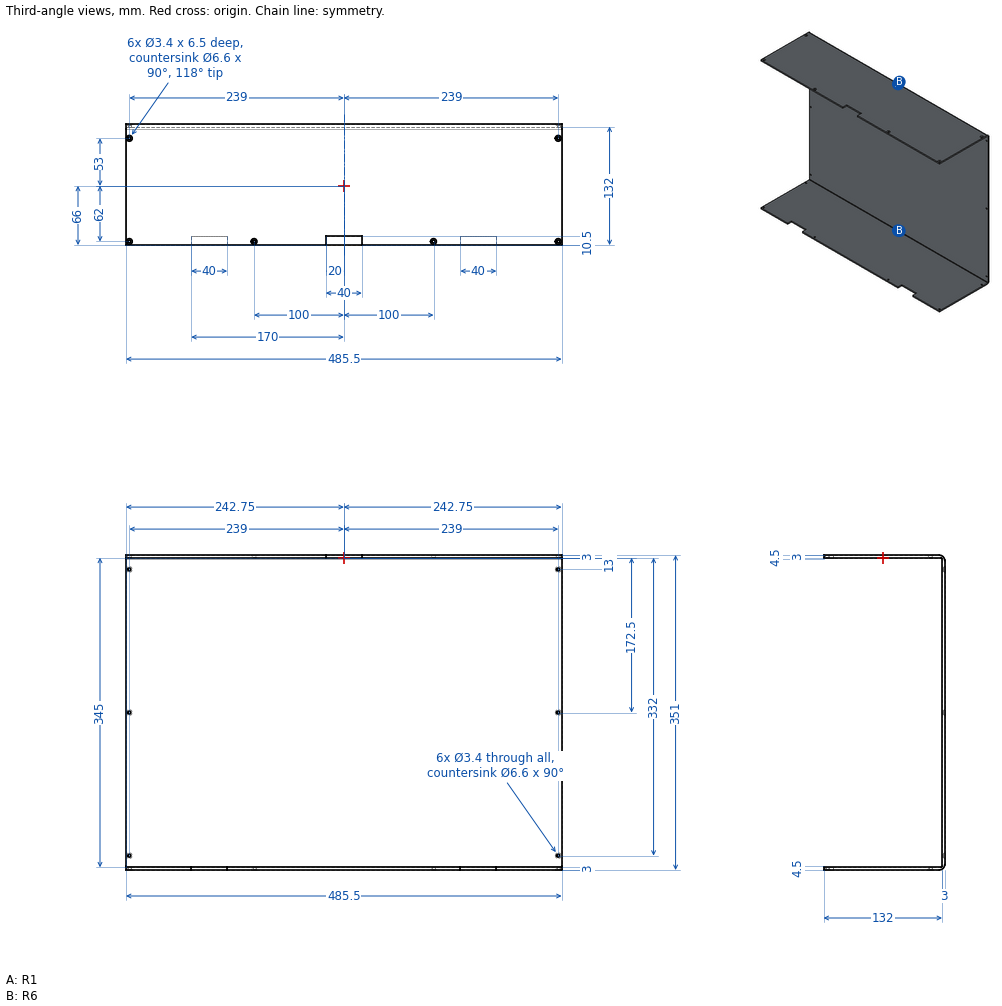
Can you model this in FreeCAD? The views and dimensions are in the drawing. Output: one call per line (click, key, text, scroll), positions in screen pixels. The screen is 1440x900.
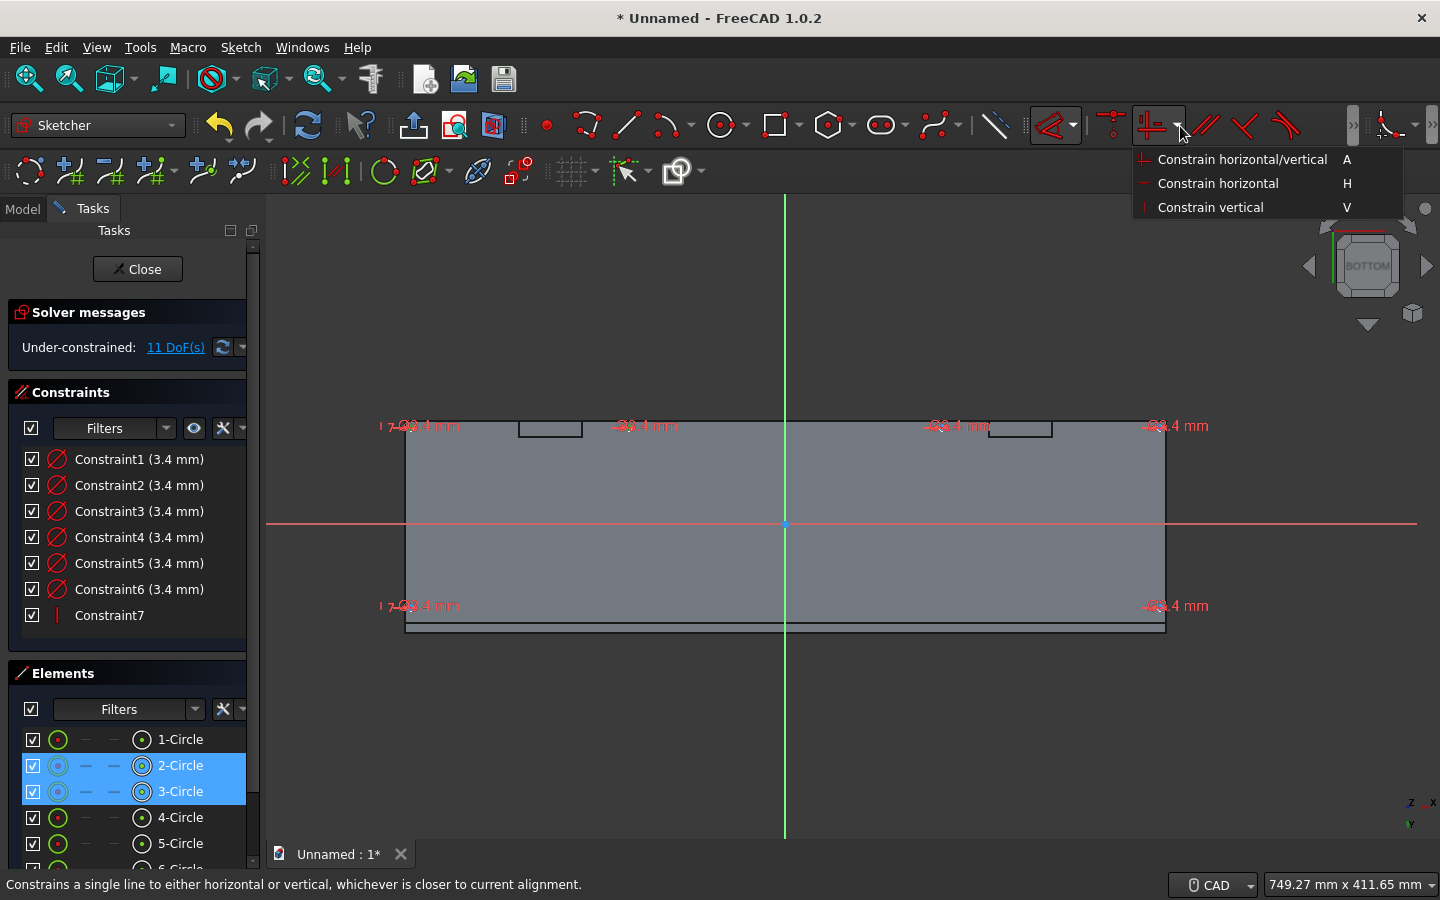
click(1268, 183)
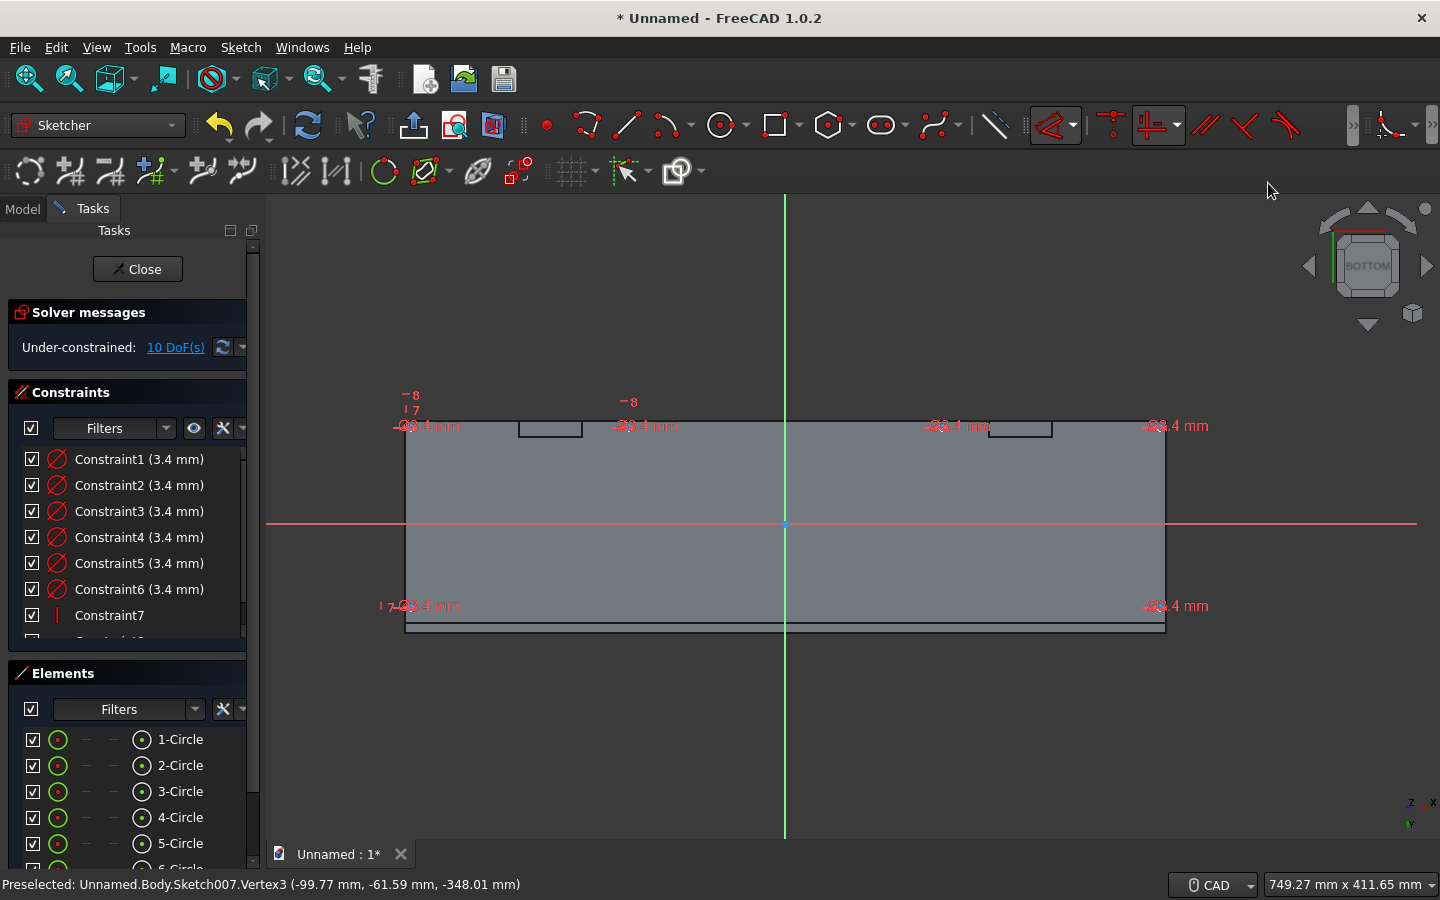
click(629, 428)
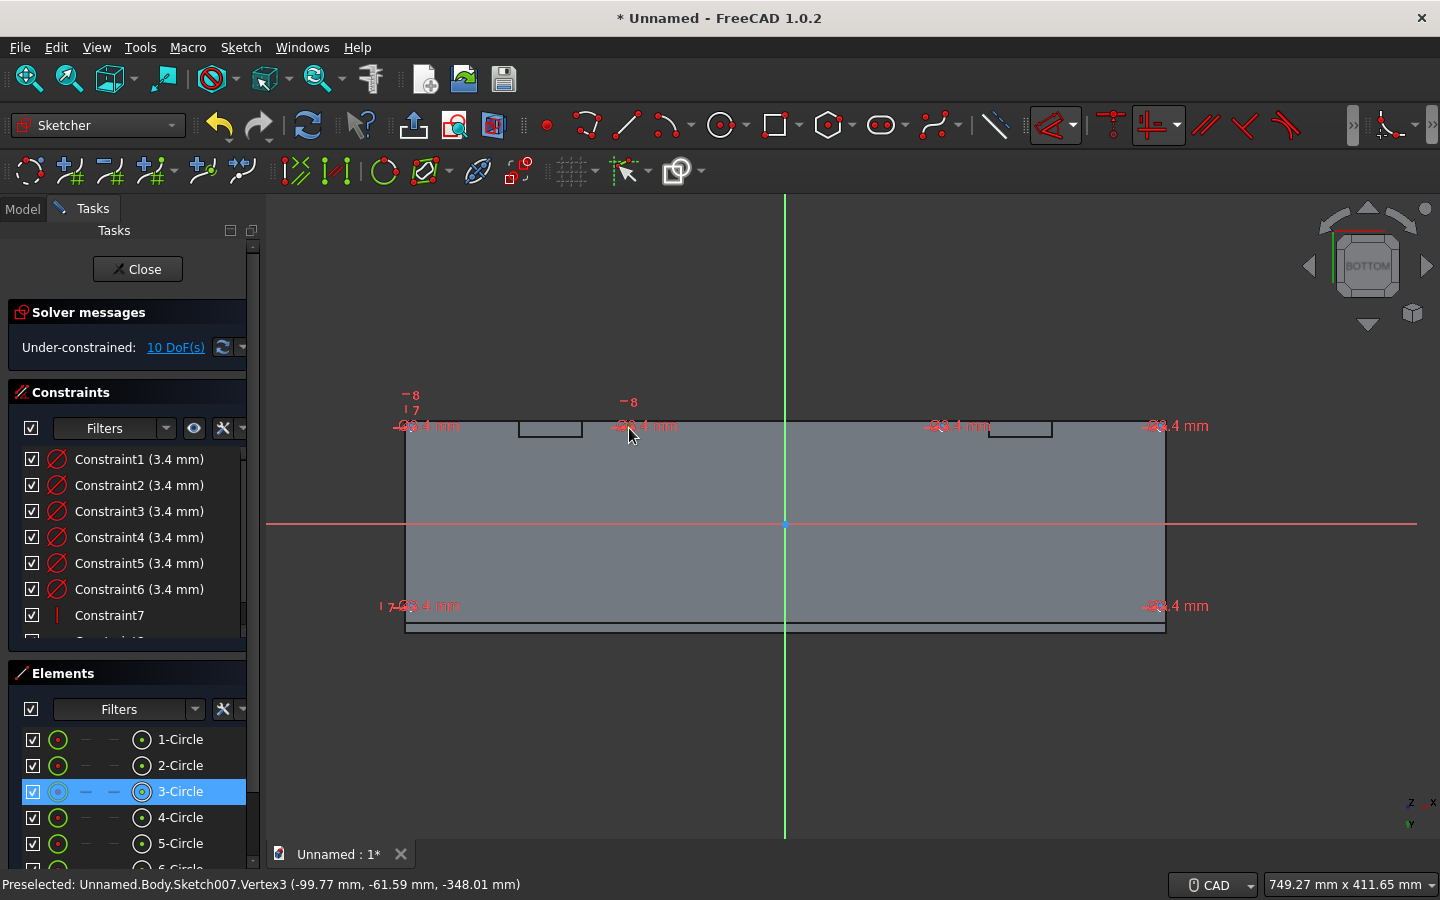
click(942, 428)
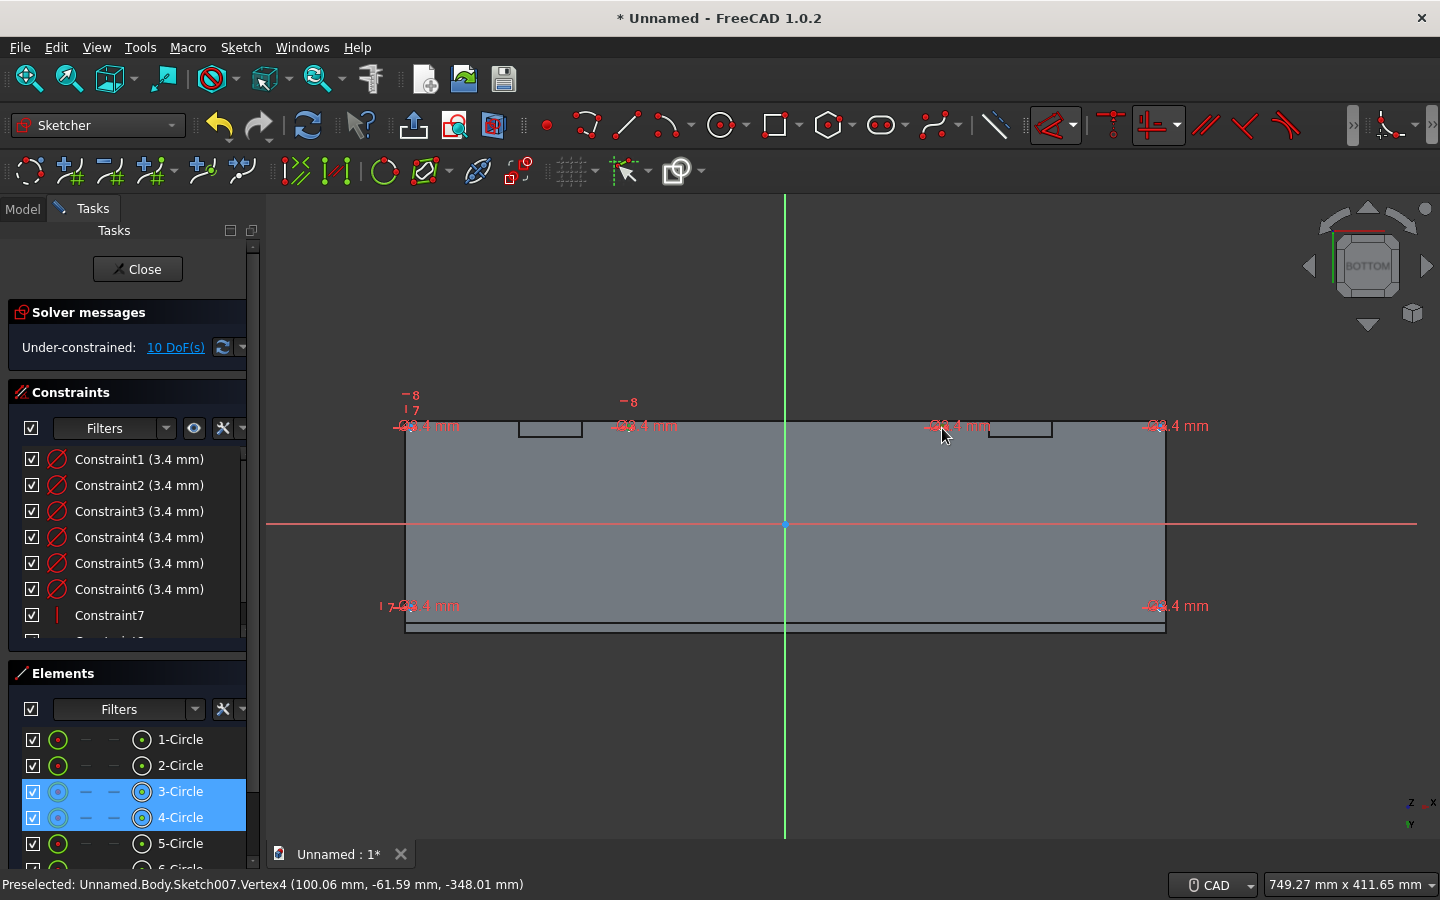
click(1180, 126)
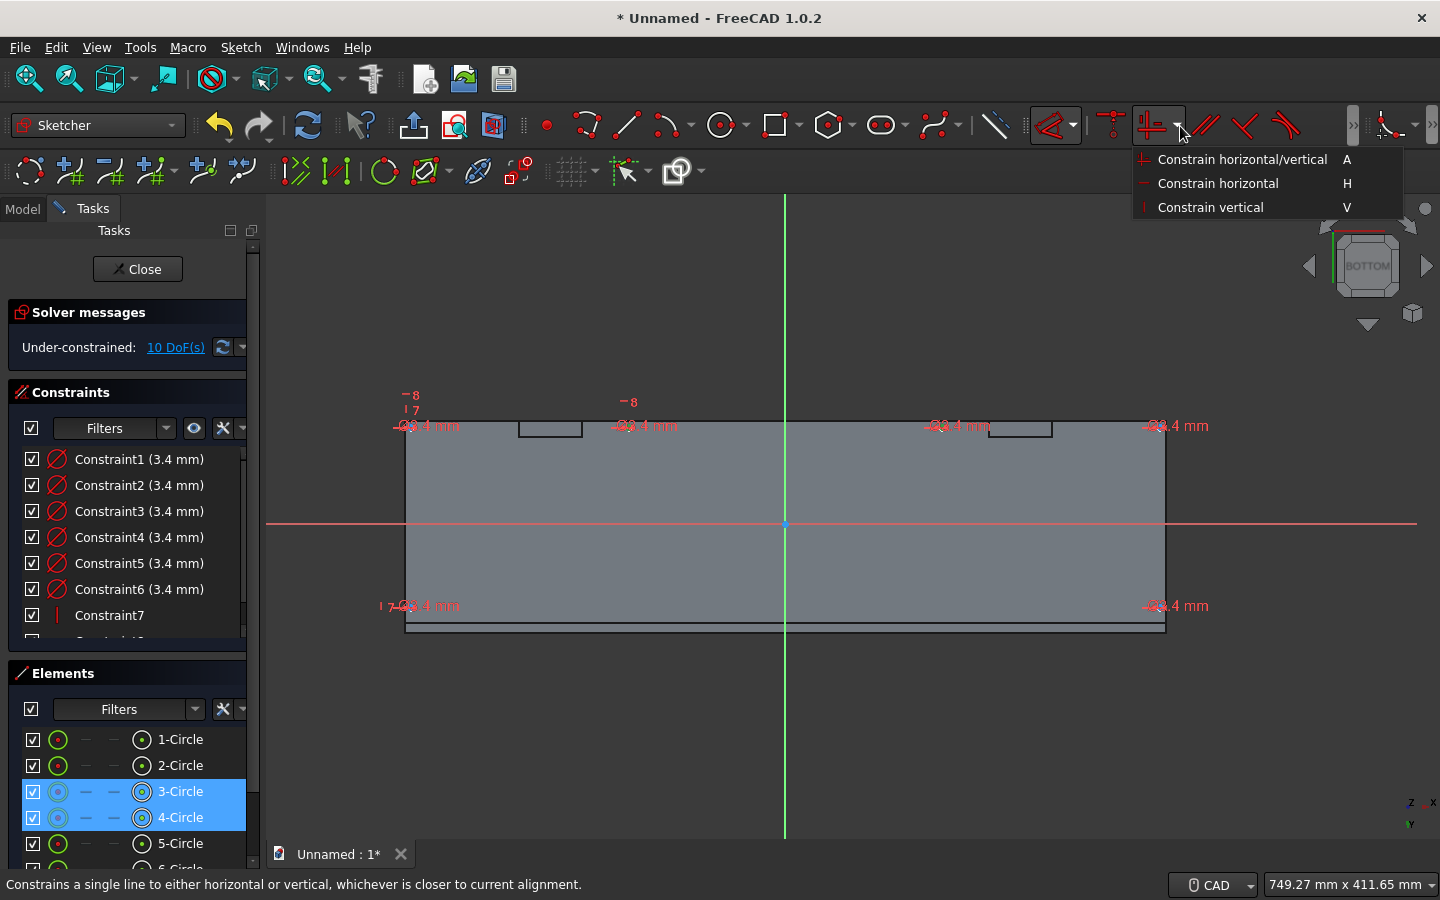
click(1268, 183)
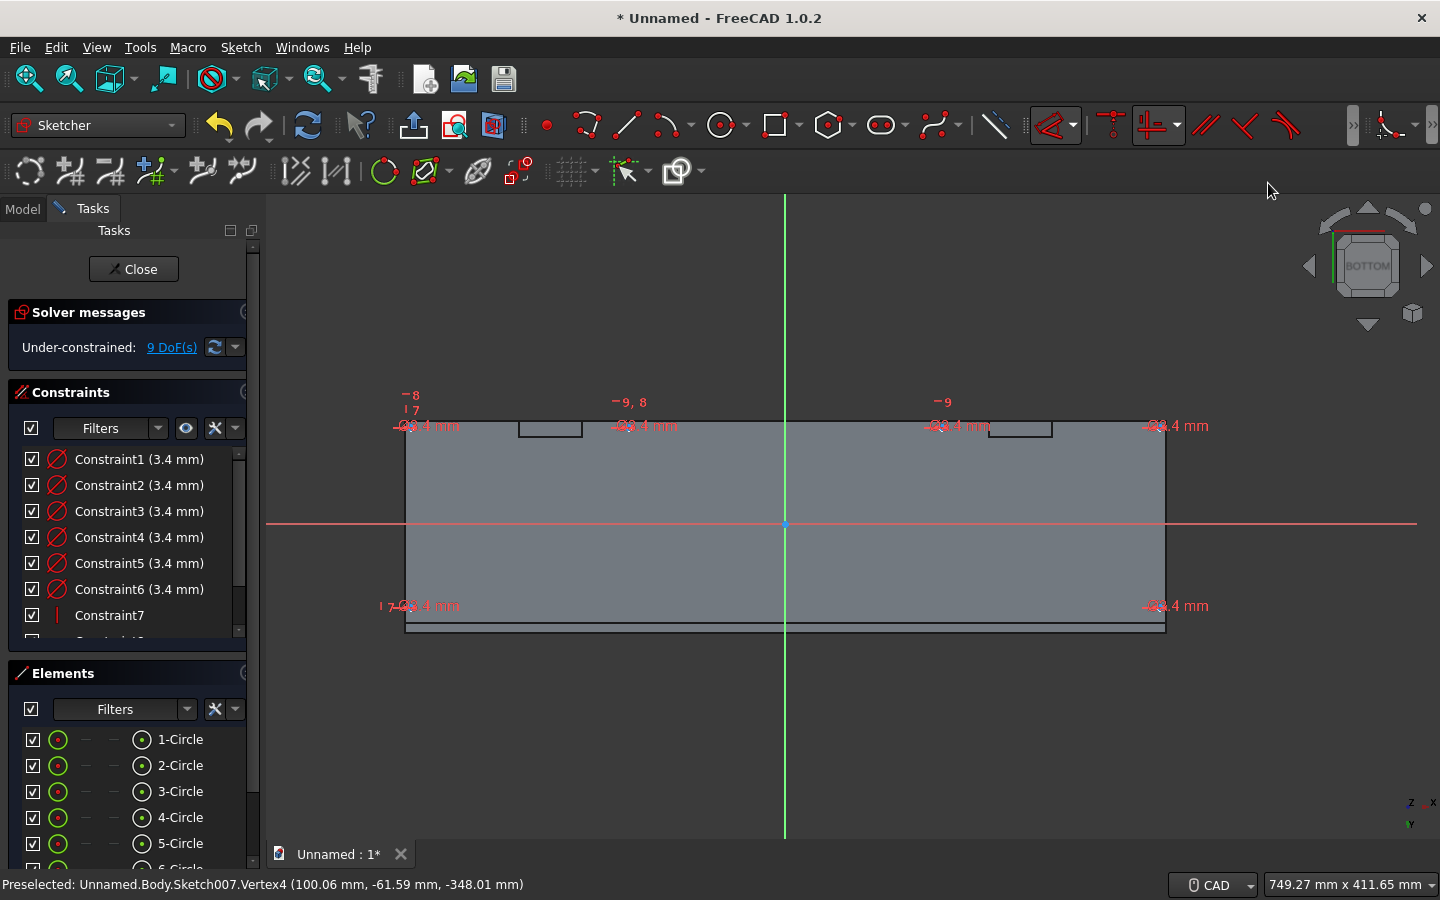
click(942, 428)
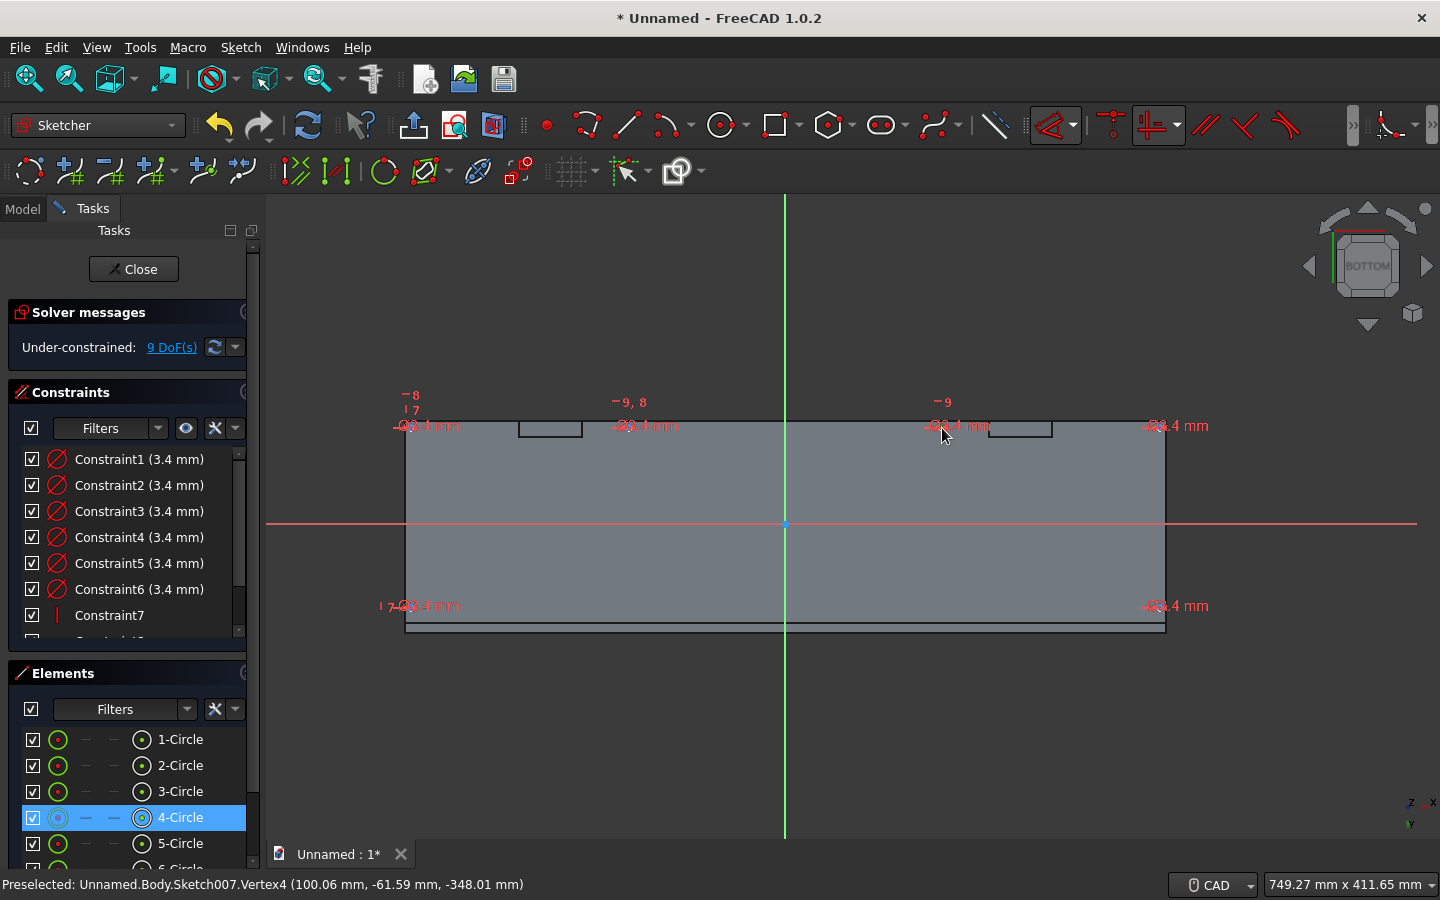
click(1160, 428)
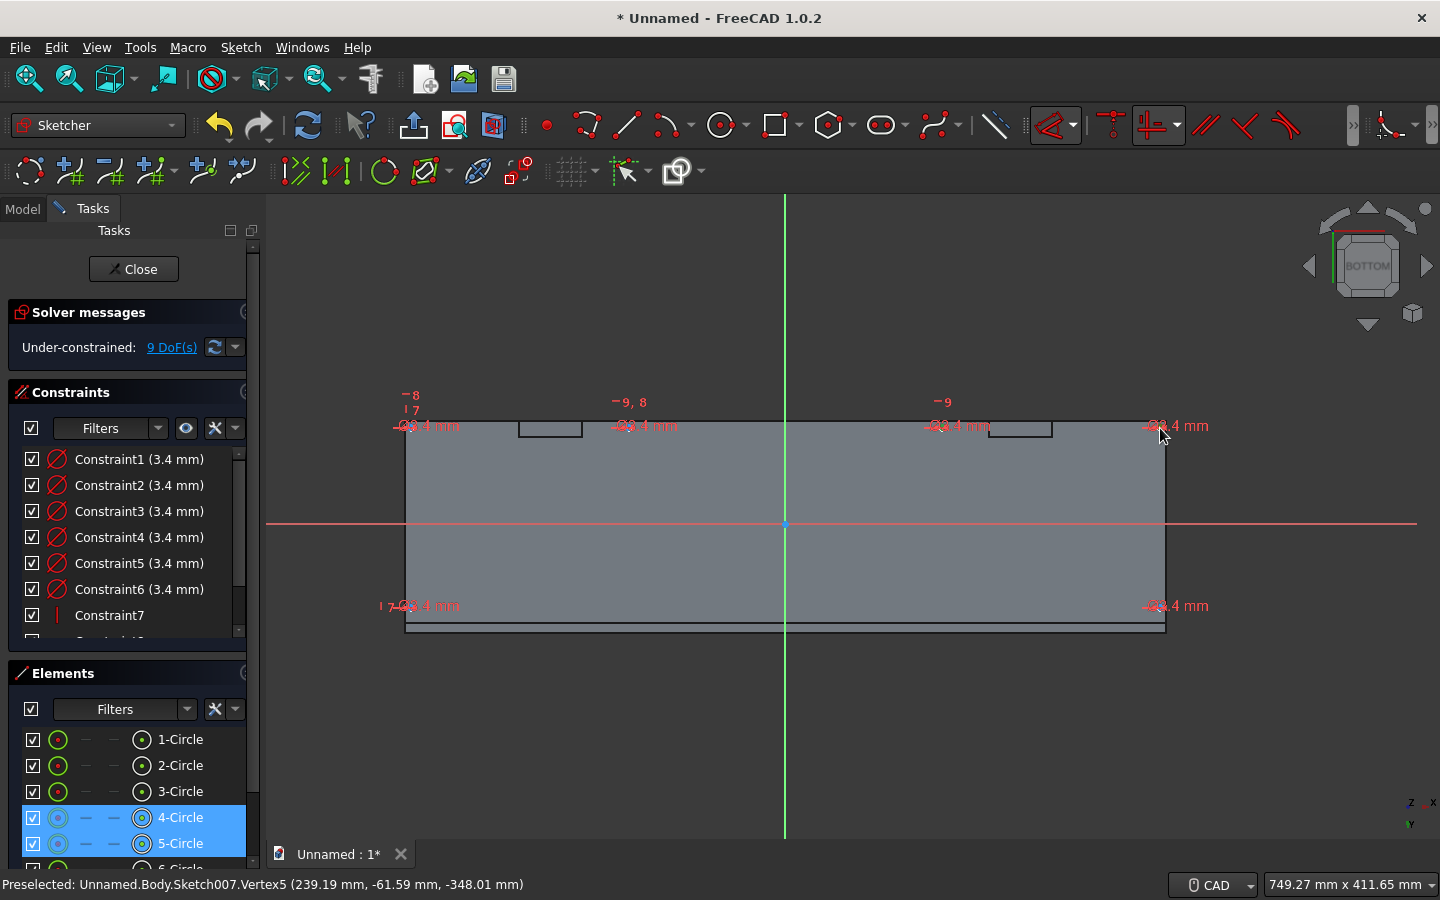
click(1180, 126)